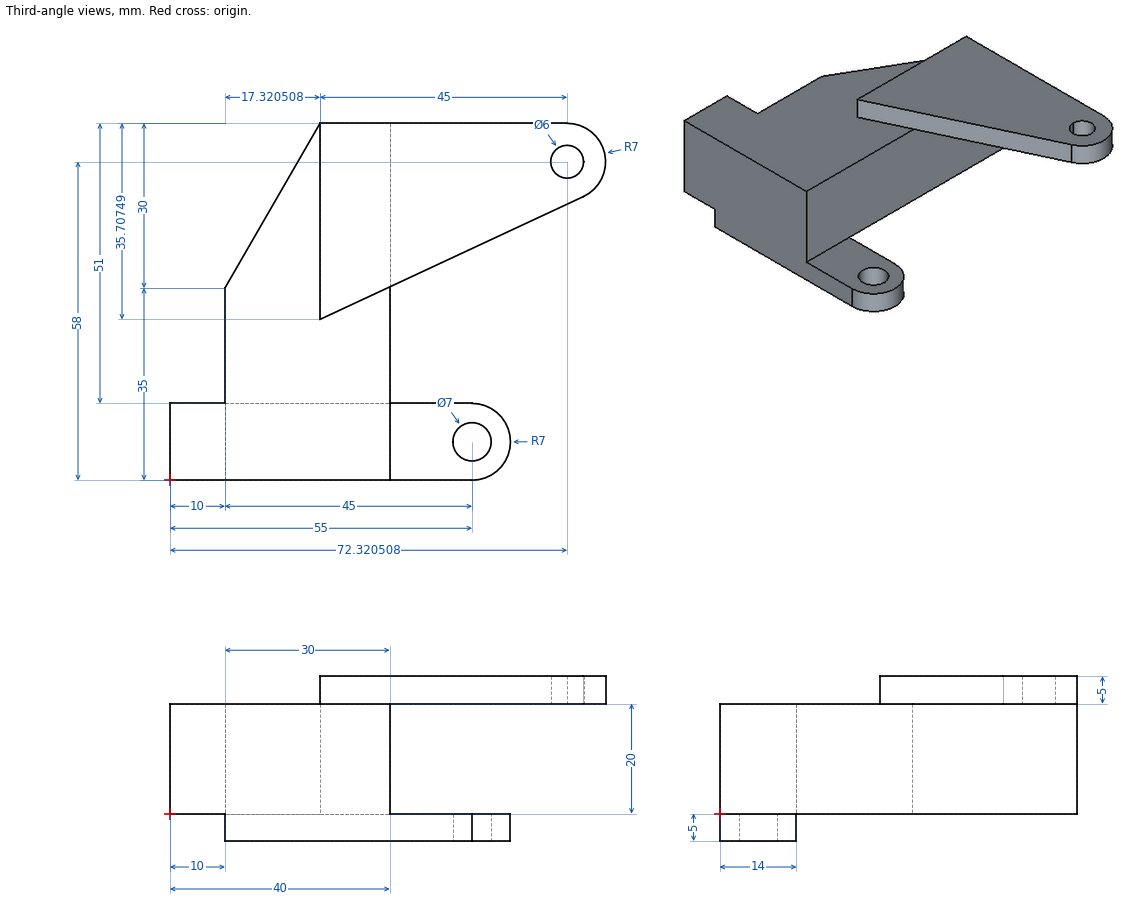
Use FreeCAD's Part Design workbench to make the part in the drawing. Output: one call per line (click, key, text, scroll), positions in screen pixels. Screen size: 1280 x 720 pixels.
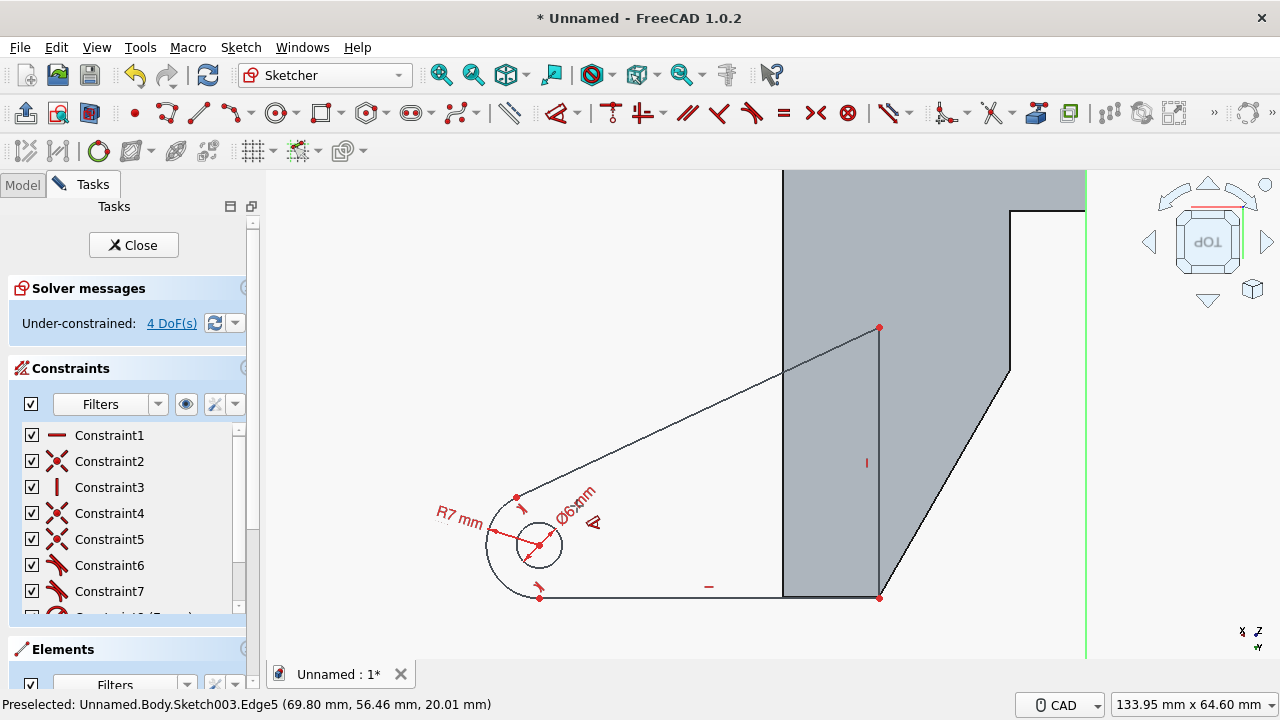
click(641, 598)
click(709, 564)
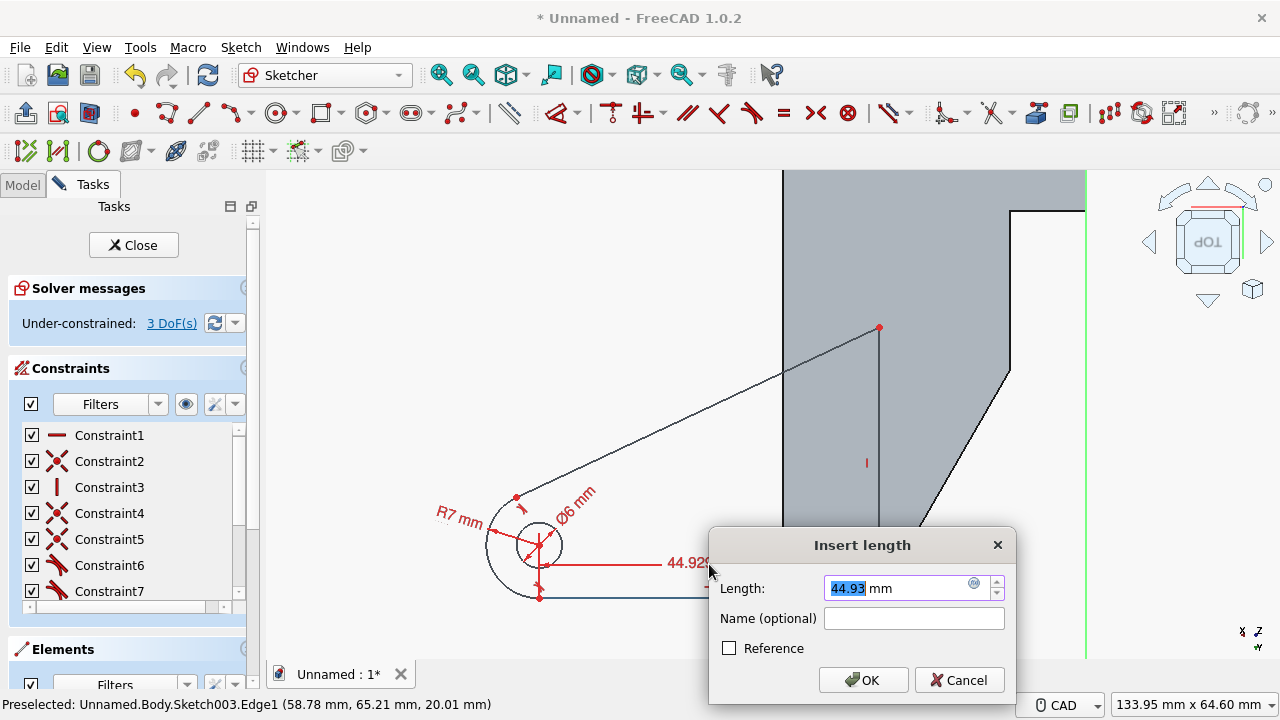
text(45)
key(Return)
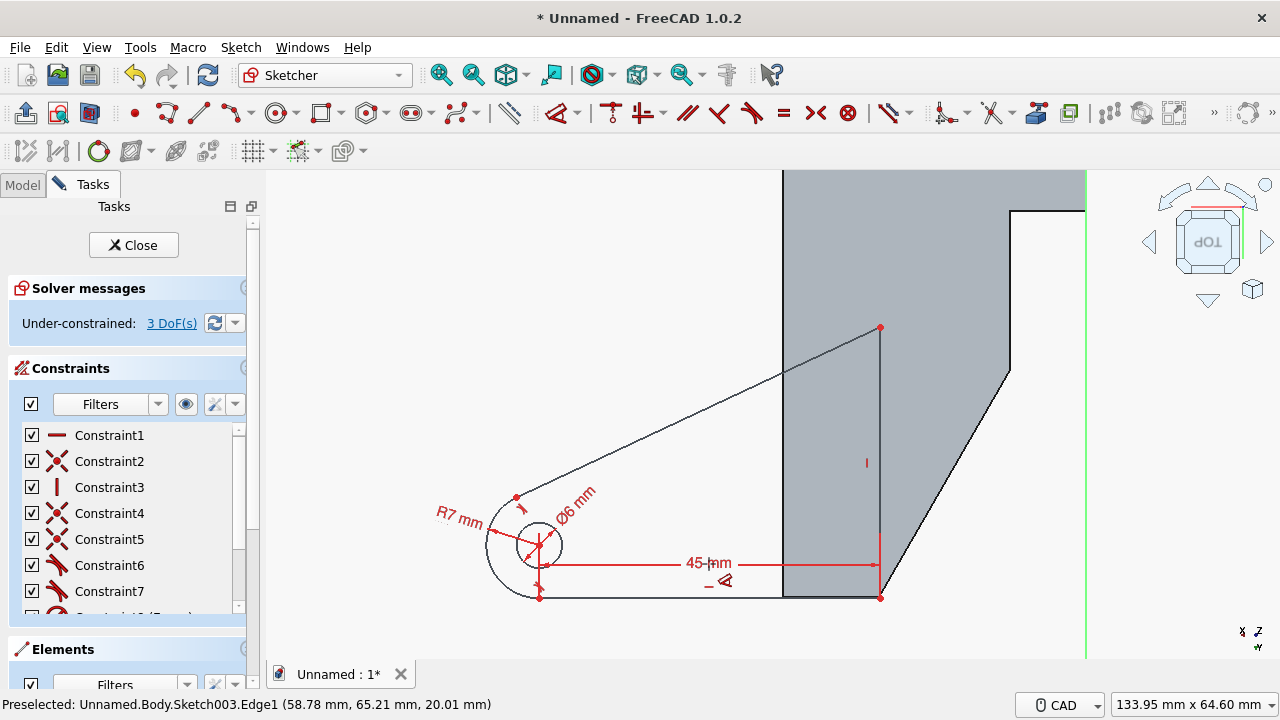
click(539, 545)
click(505, 372)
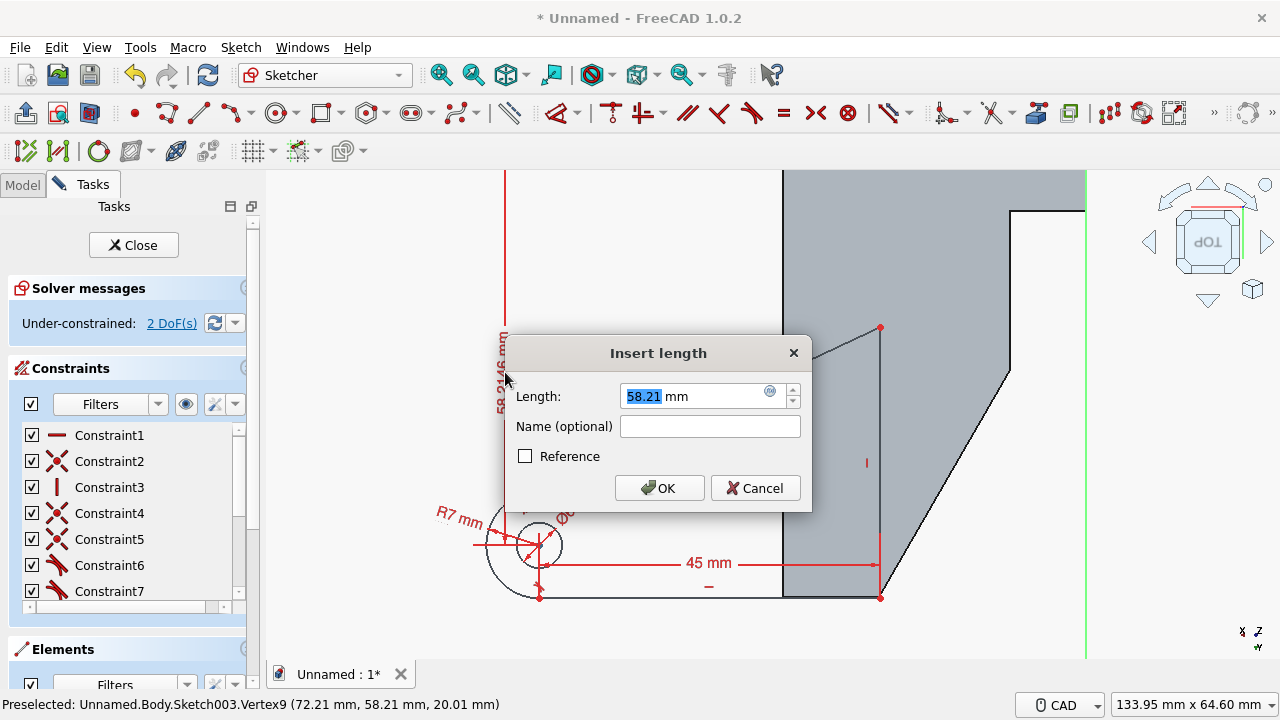
text(58)
key(Return)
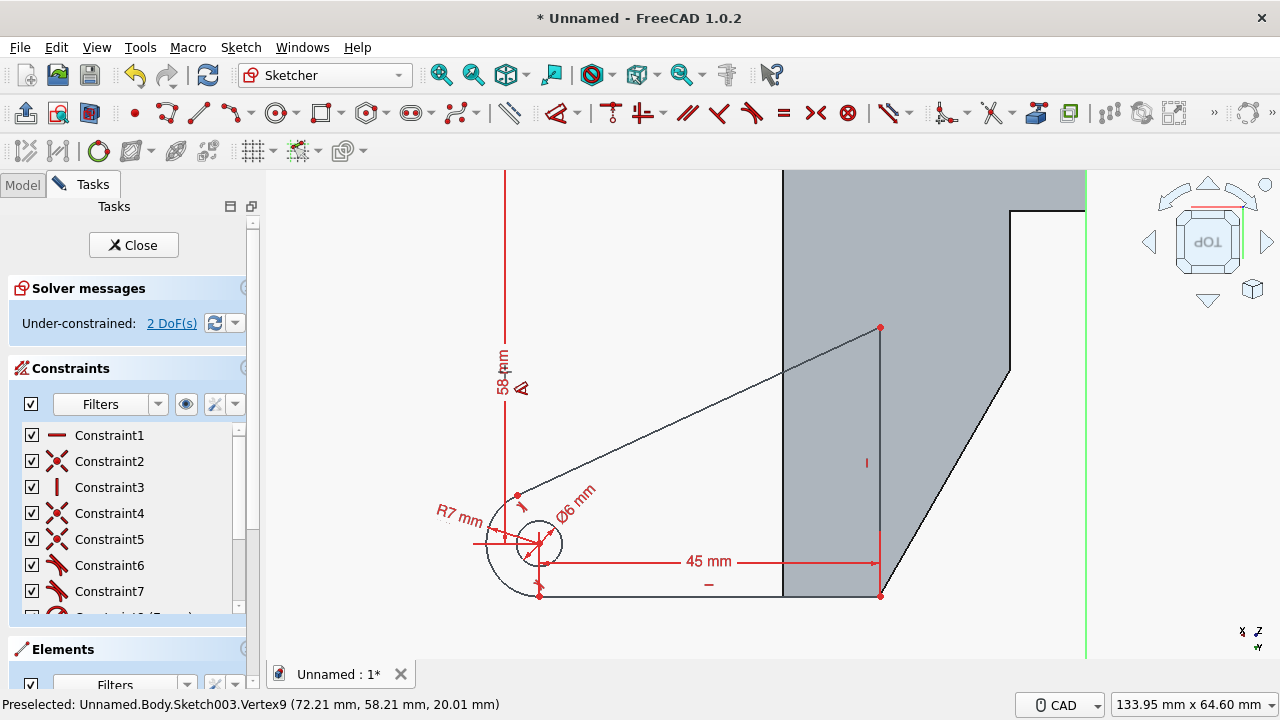
click(880, 516)
click(914, 462)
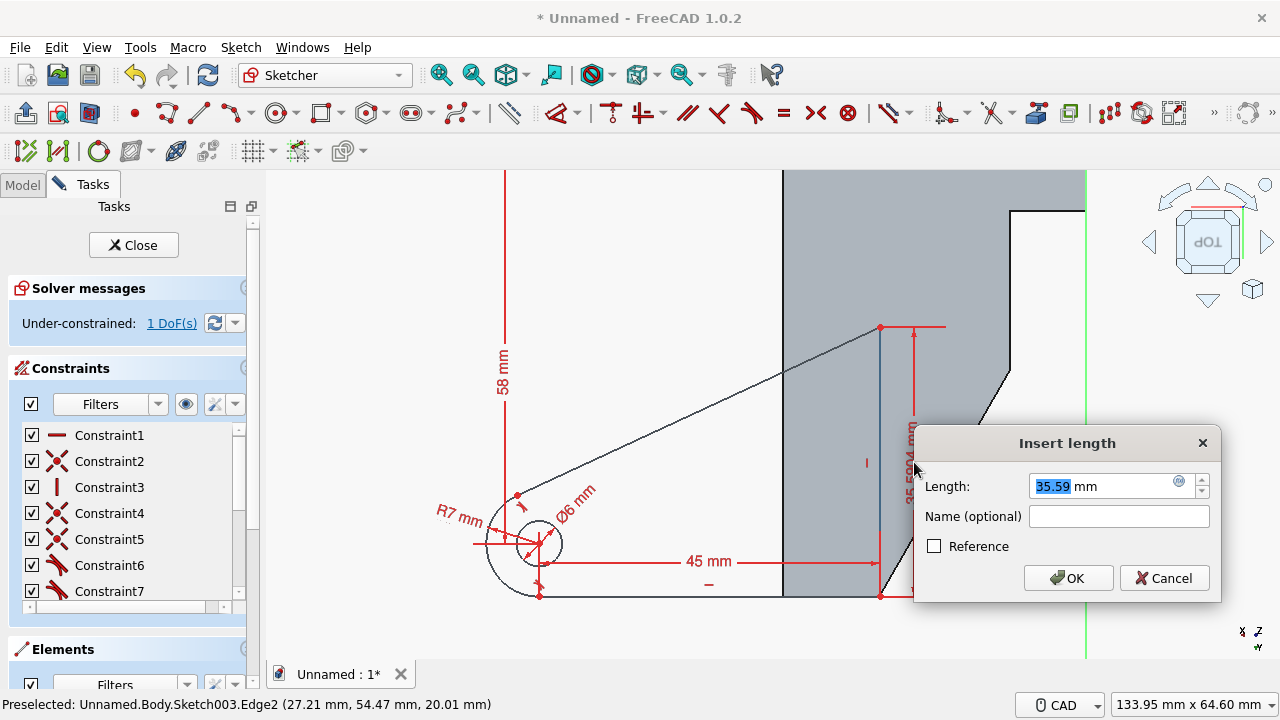
text(35.70749)
key(Return)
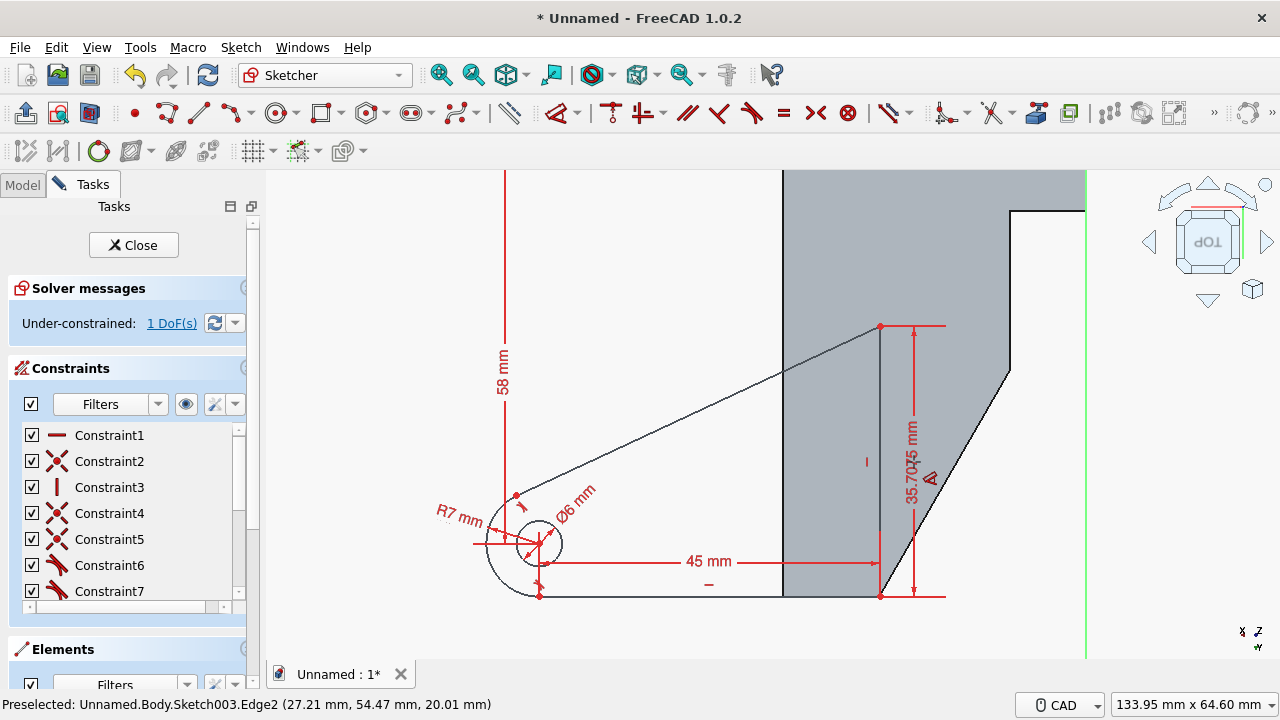
click(539, 544)
click(813, 578)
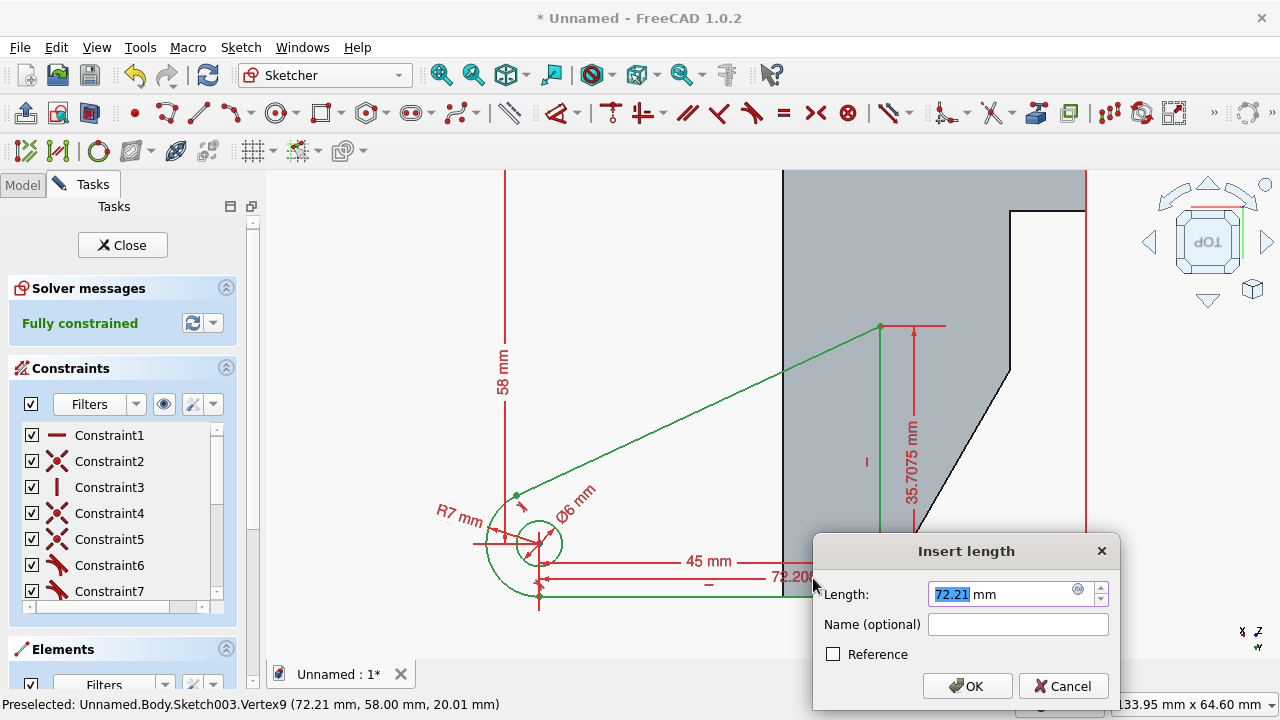
text(72.320508)
key(Return)
key(Escape)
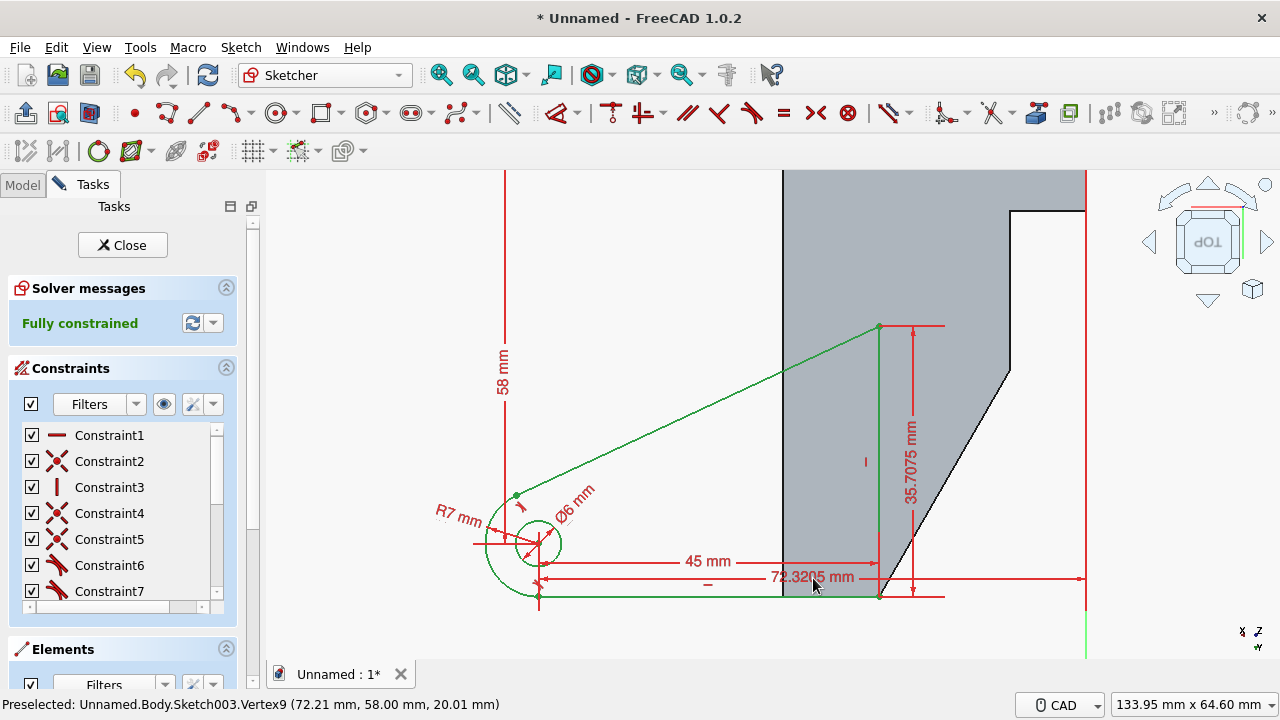
click(123, 245)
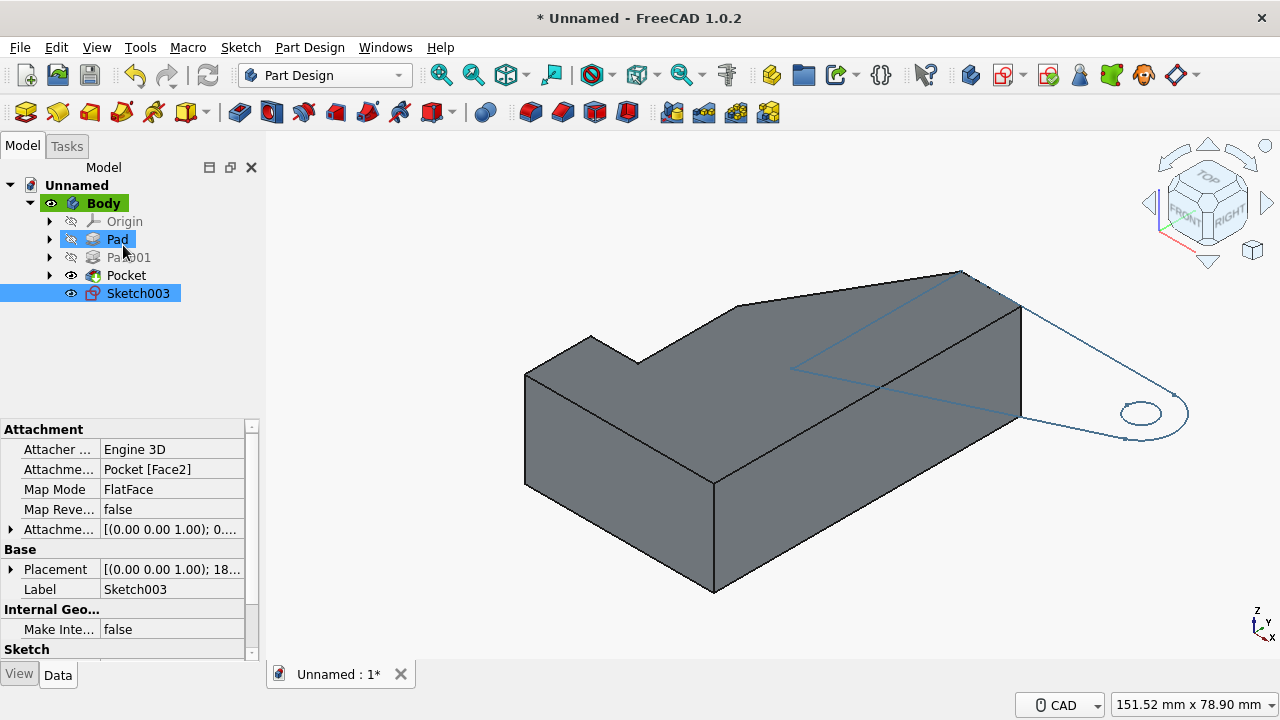
click(26, 112)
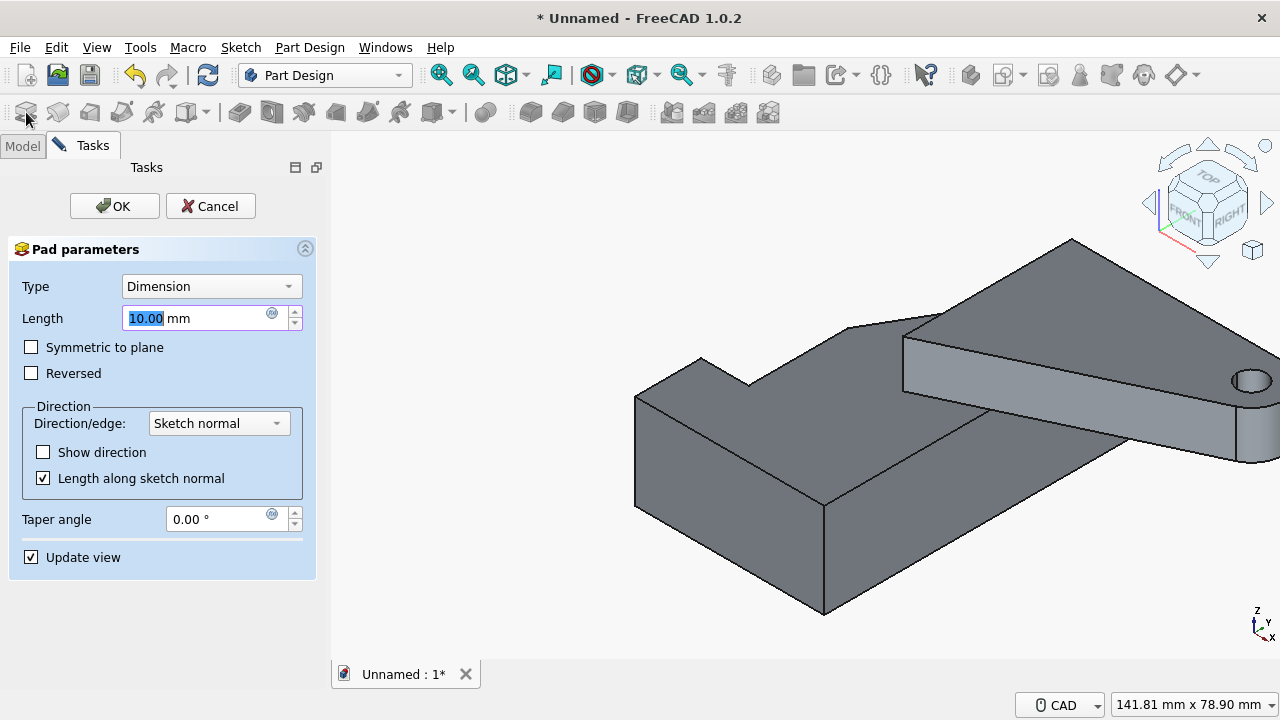
text(5)
key(Tab)